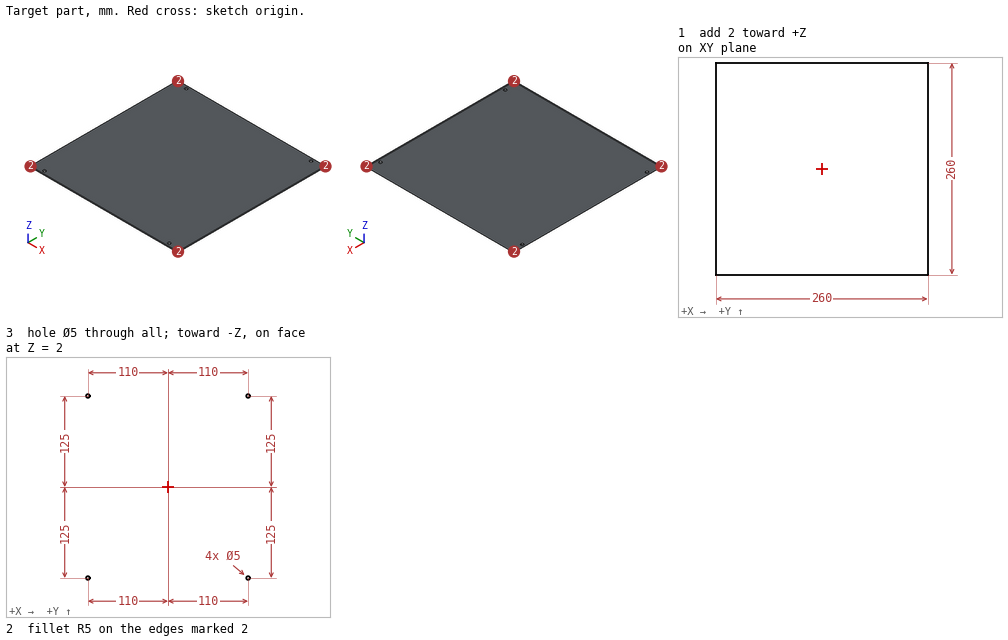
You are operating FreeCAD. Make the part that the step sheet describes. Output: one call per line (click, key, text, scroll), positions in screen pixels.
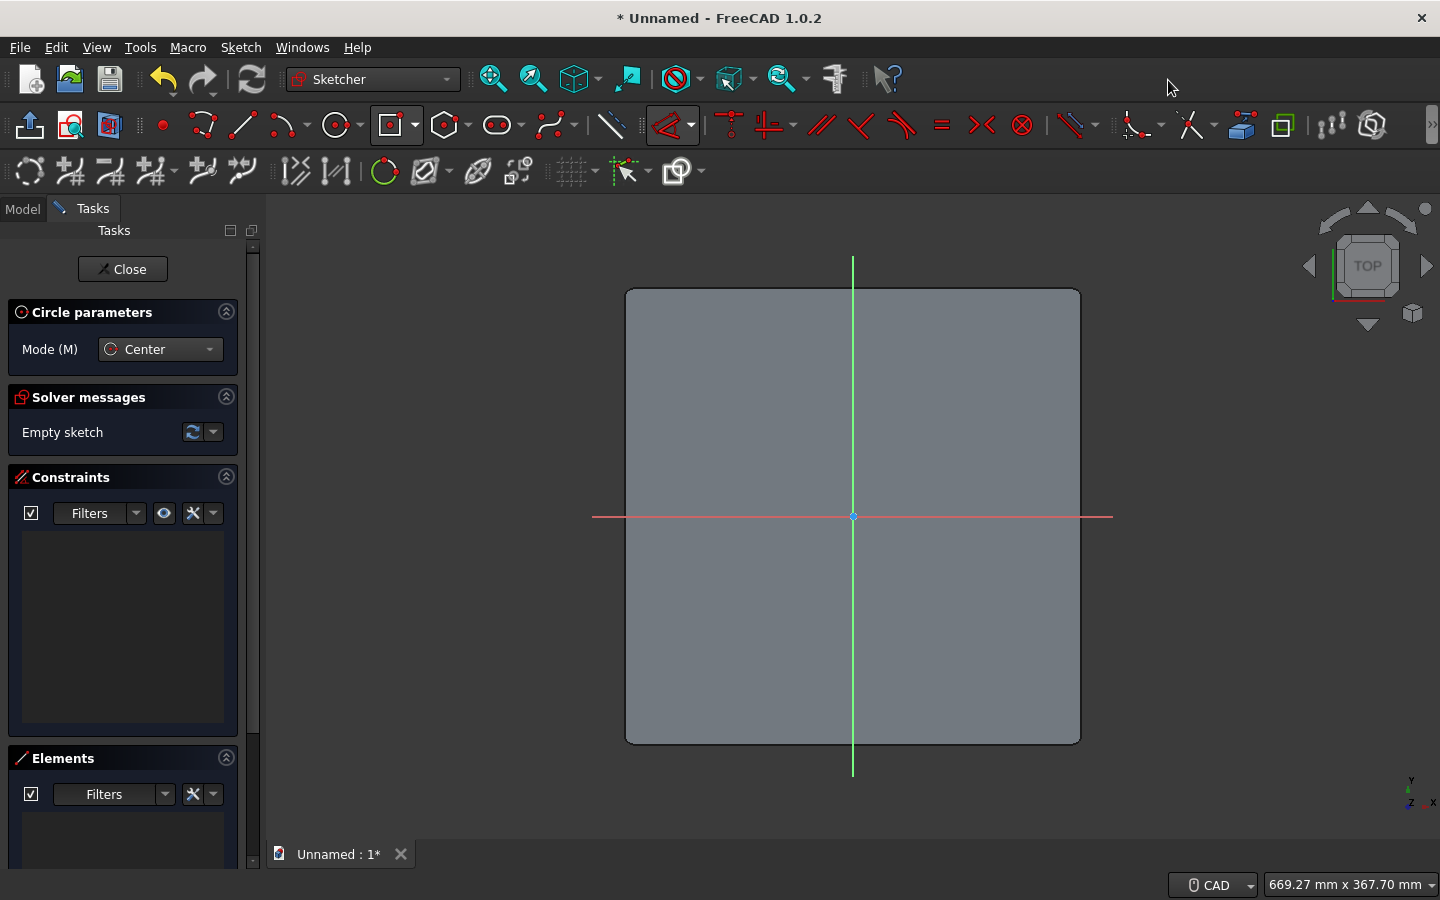
scroll(660, 297, up, 9)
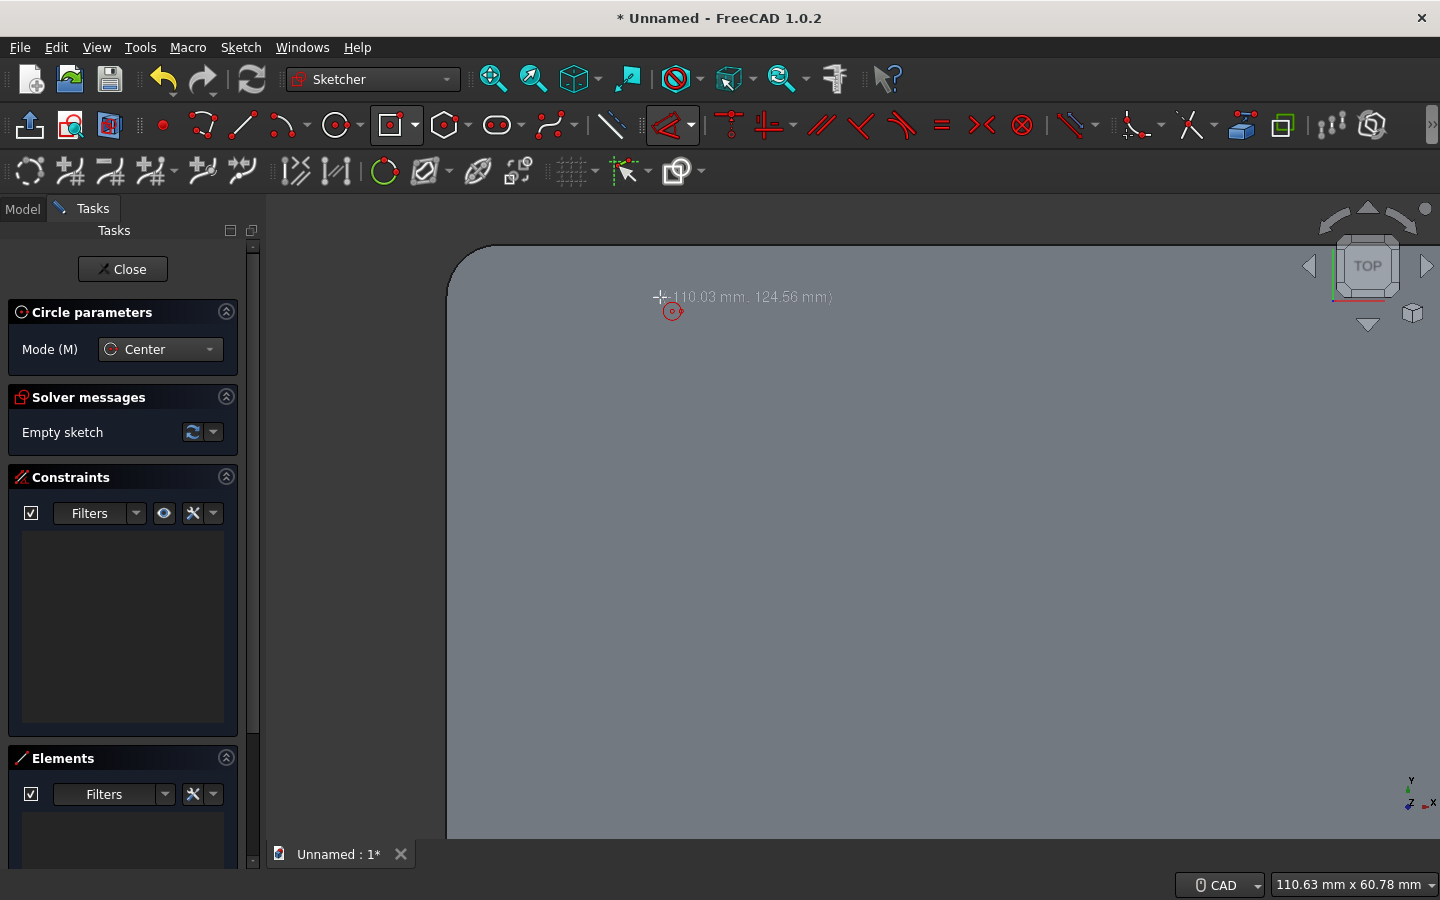
scroll(578, 297, down, 9)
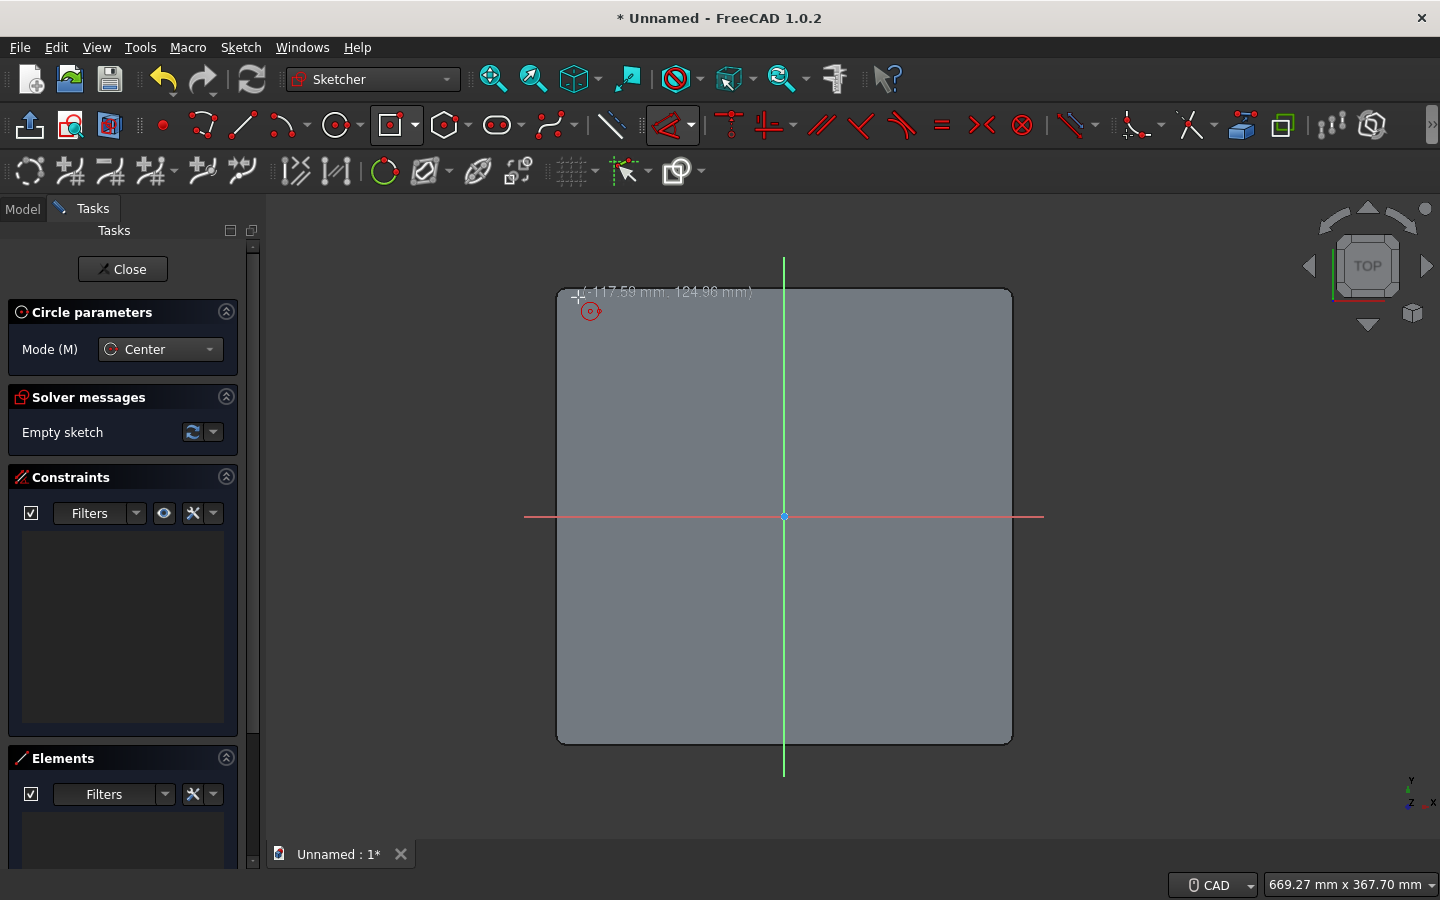
click(592, 297)
move(595, 294)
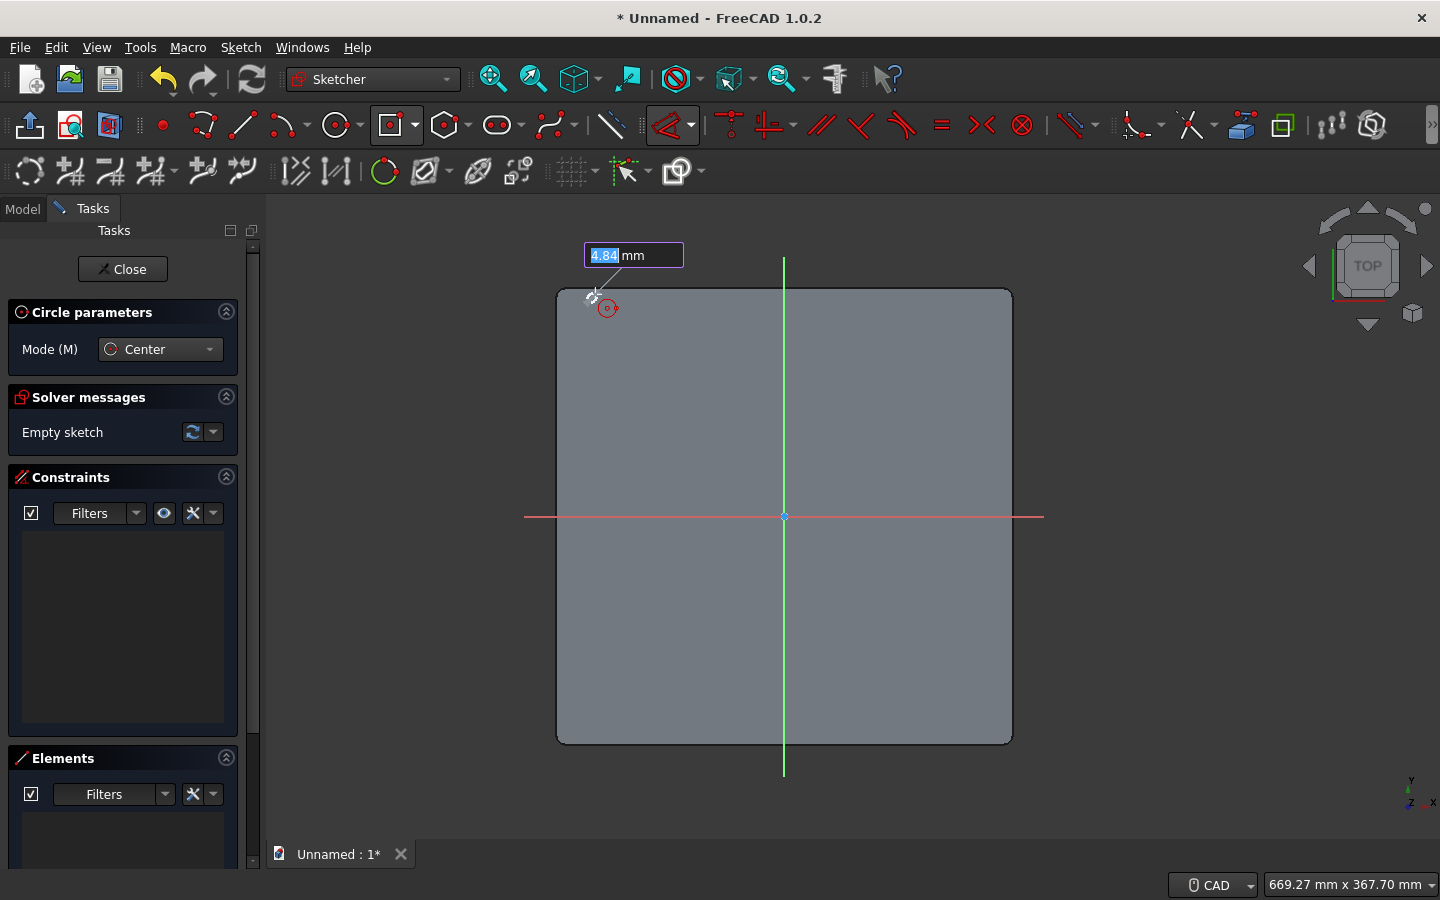
text(5)
key(Return)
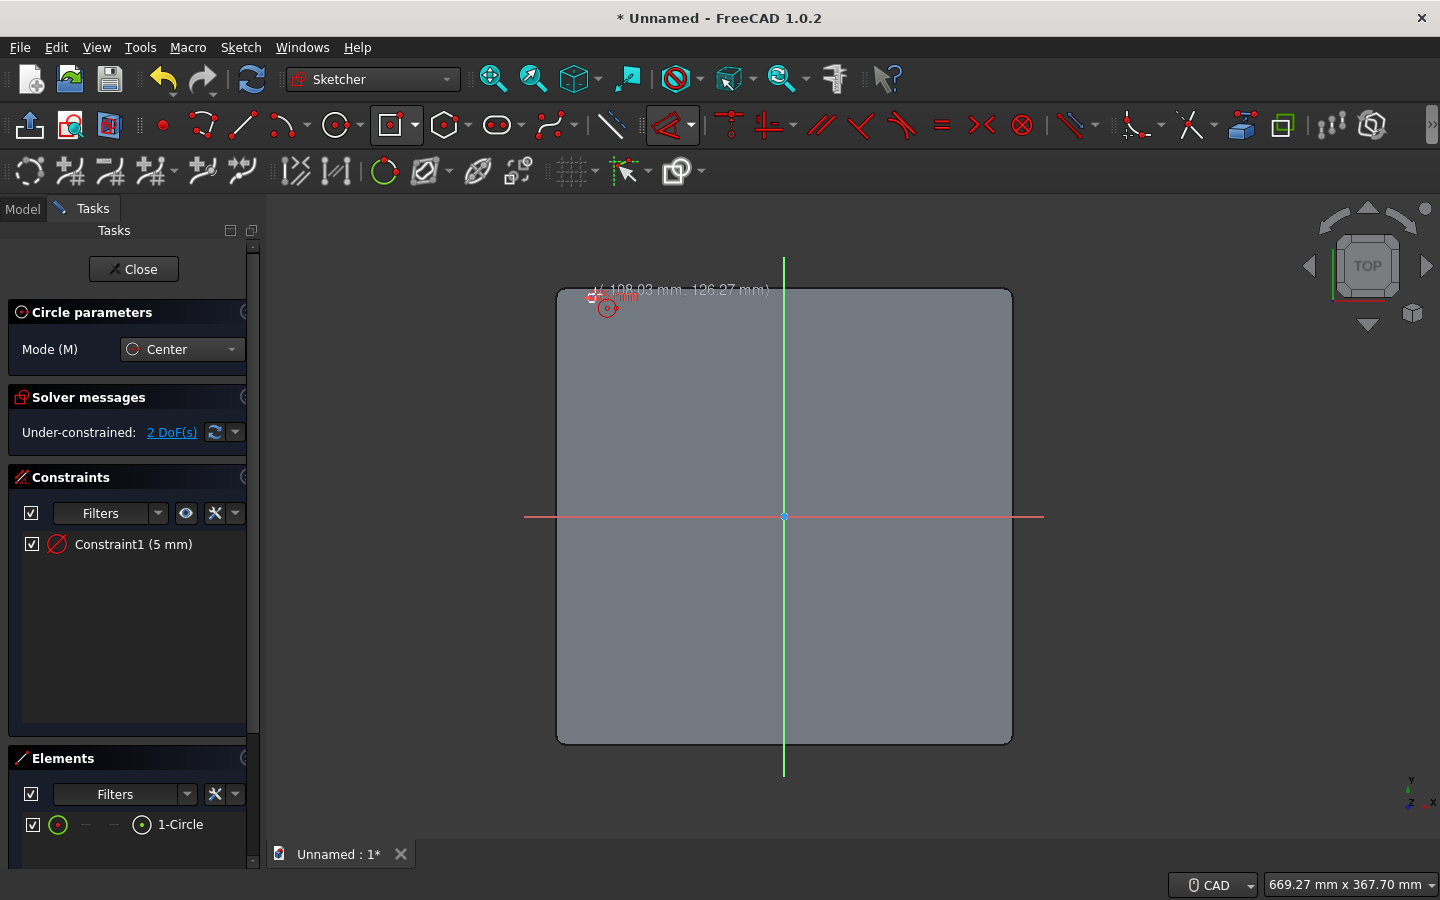
scroll(592, 736, up, 9)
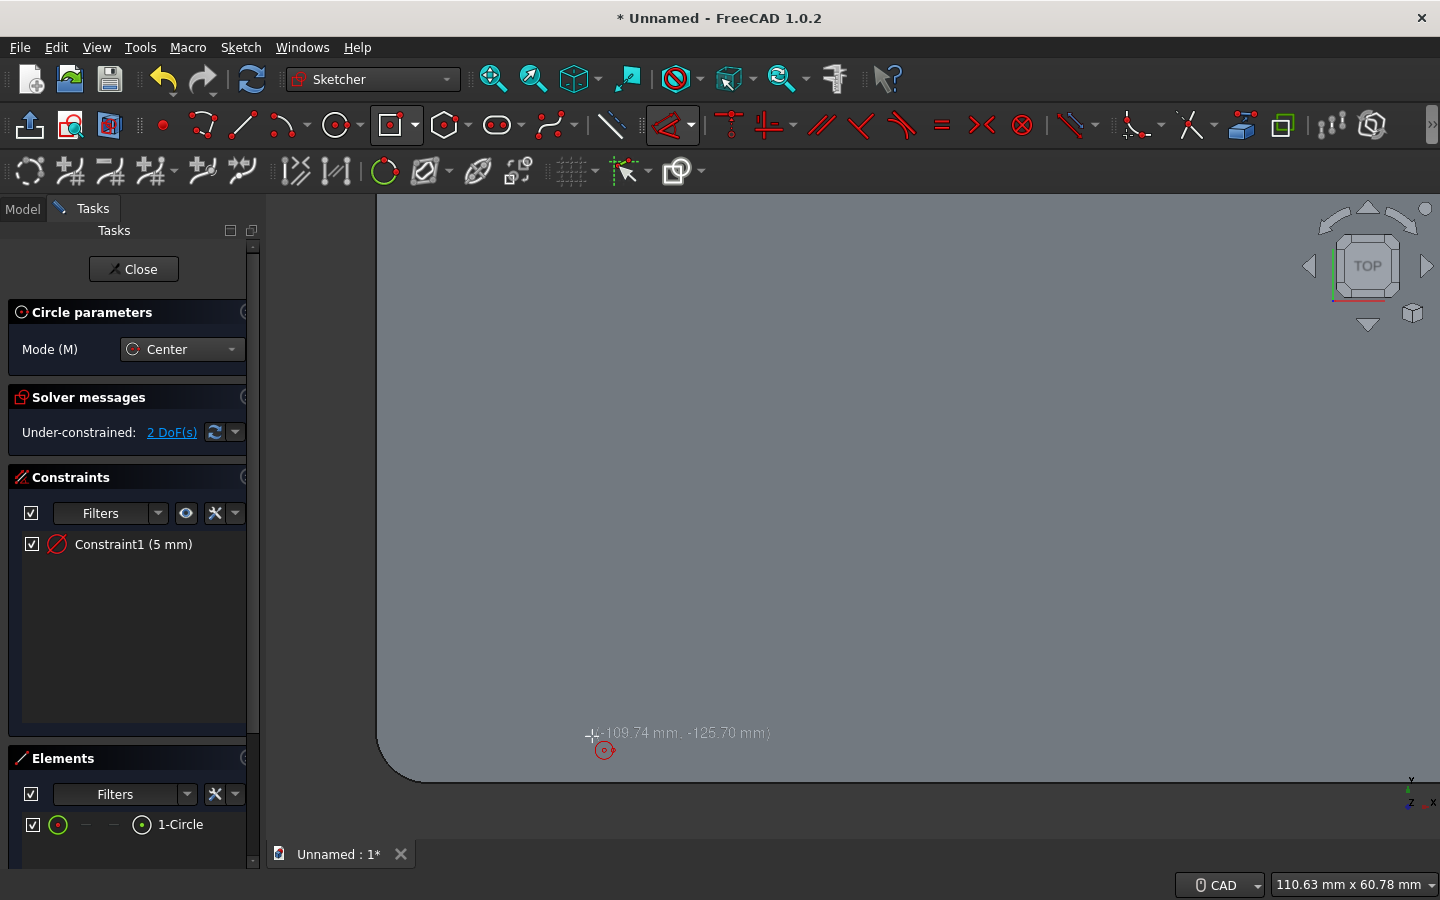
scroll(592, 737, down, 9)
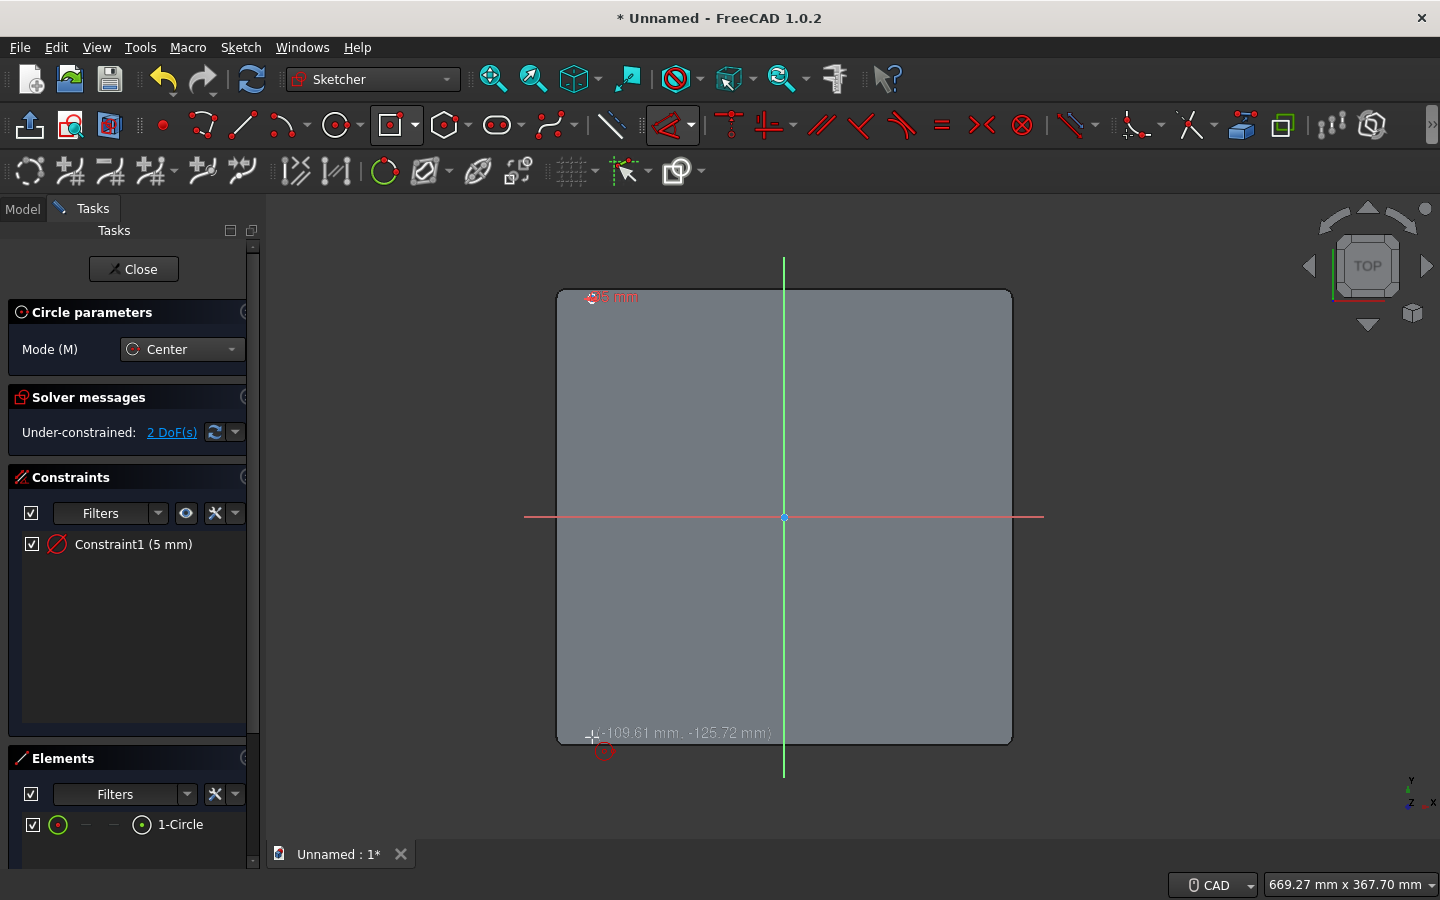
click(592, 737)
move(595, 734)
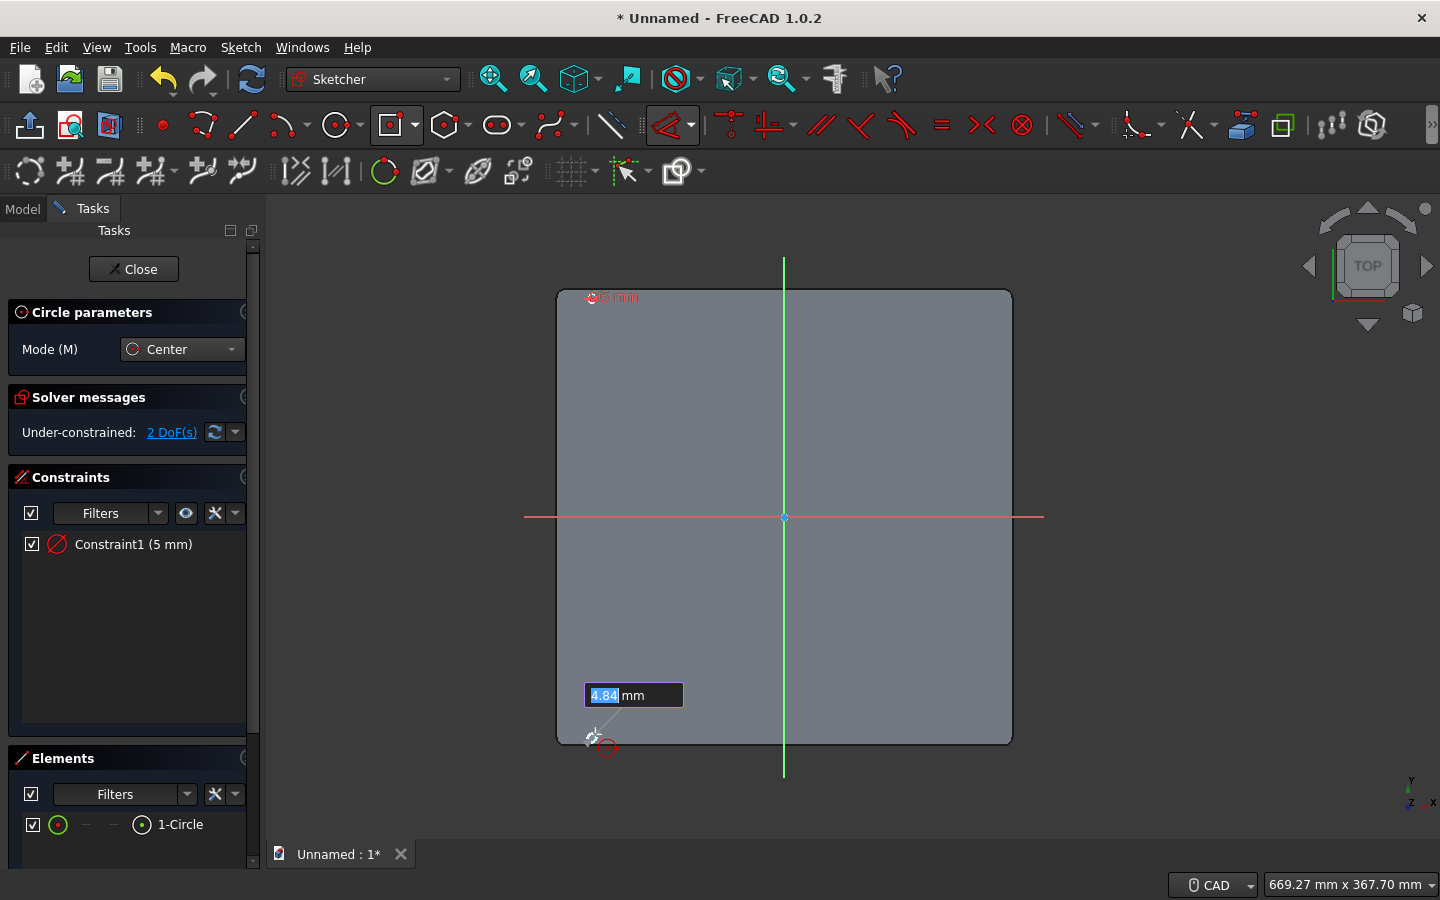
text(5)
key(Return)